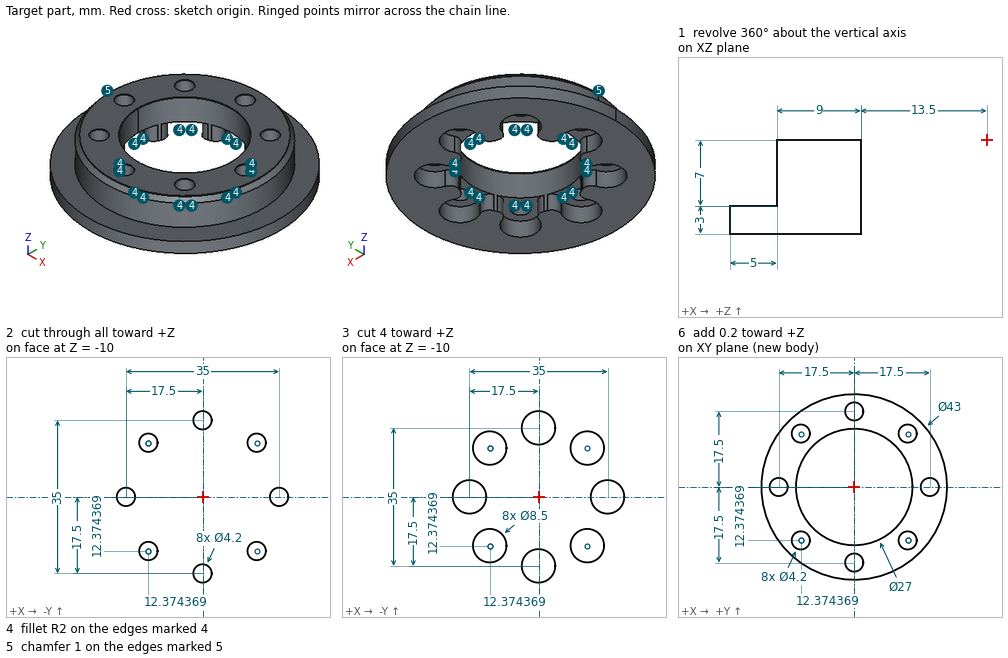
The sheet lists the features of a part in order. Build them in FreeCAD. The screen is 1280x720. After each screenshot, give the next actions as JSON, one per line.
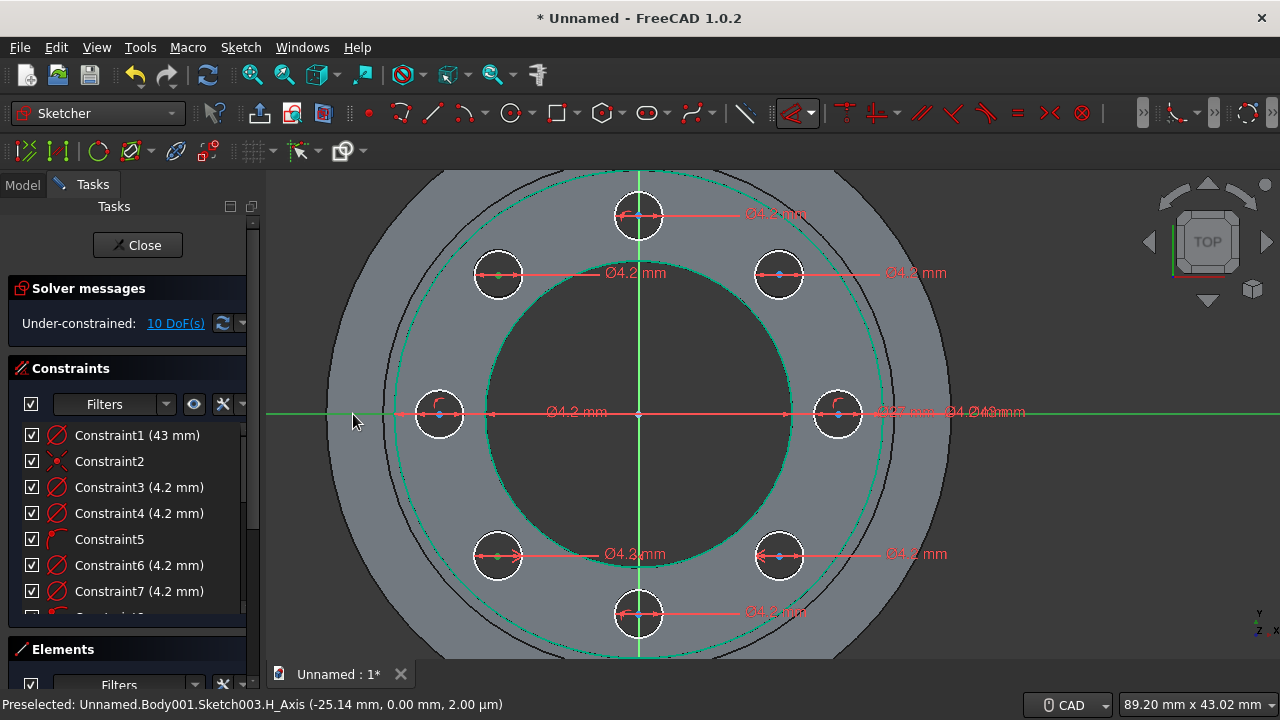
{"action": "key", "text": "s"}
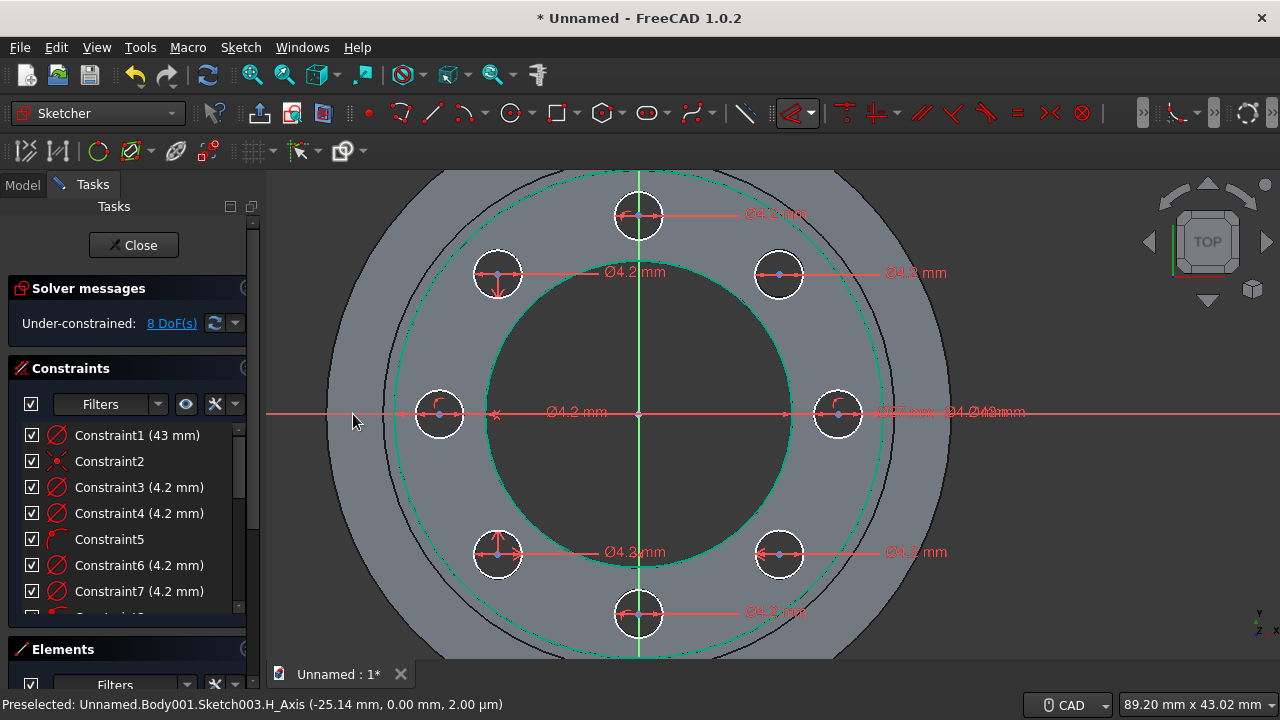
{"action": "left_click", "coordinate": [780, 554]}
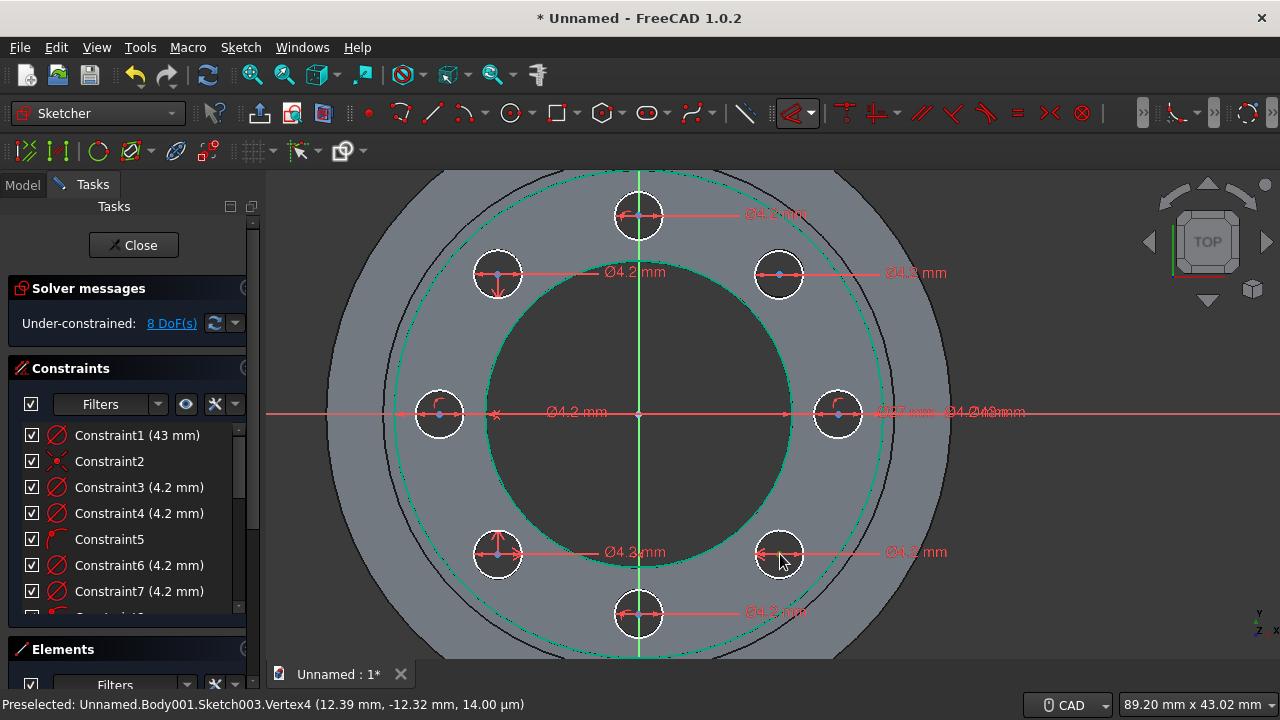
{"action": "left_click", "coordinate": [779, 275]}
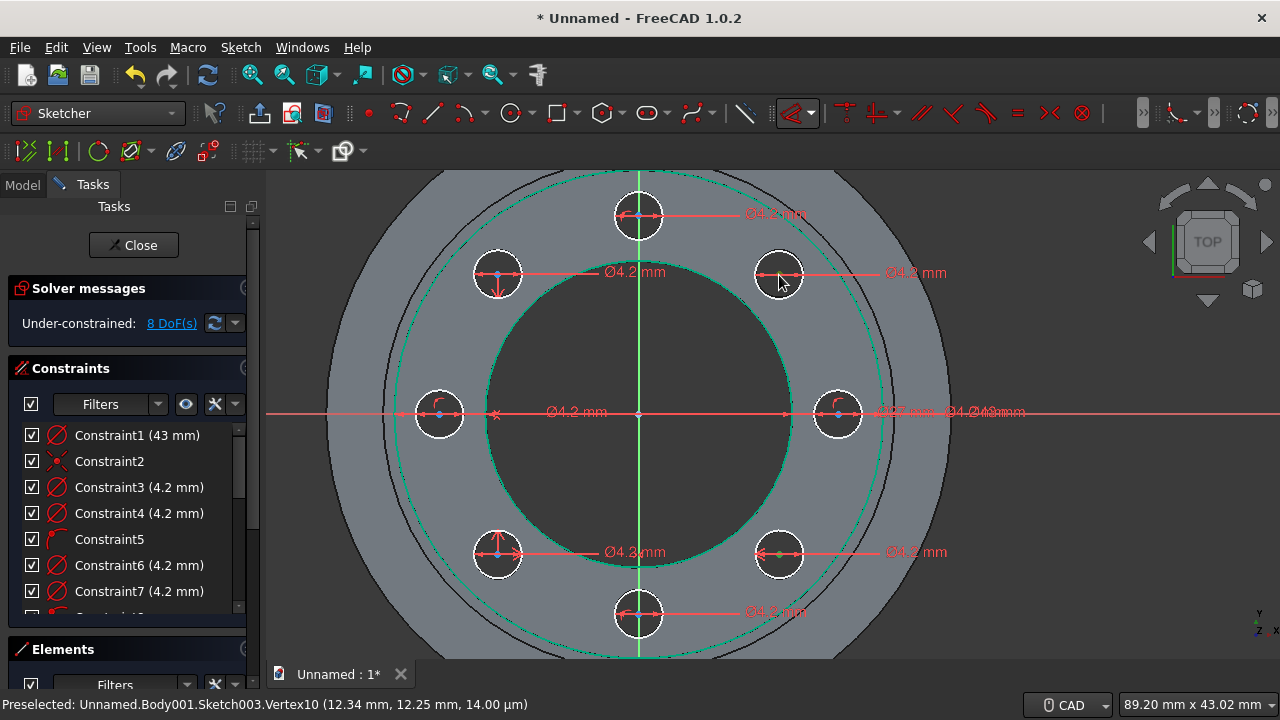
{"action": "left_click", "coordinate": [353, 414]}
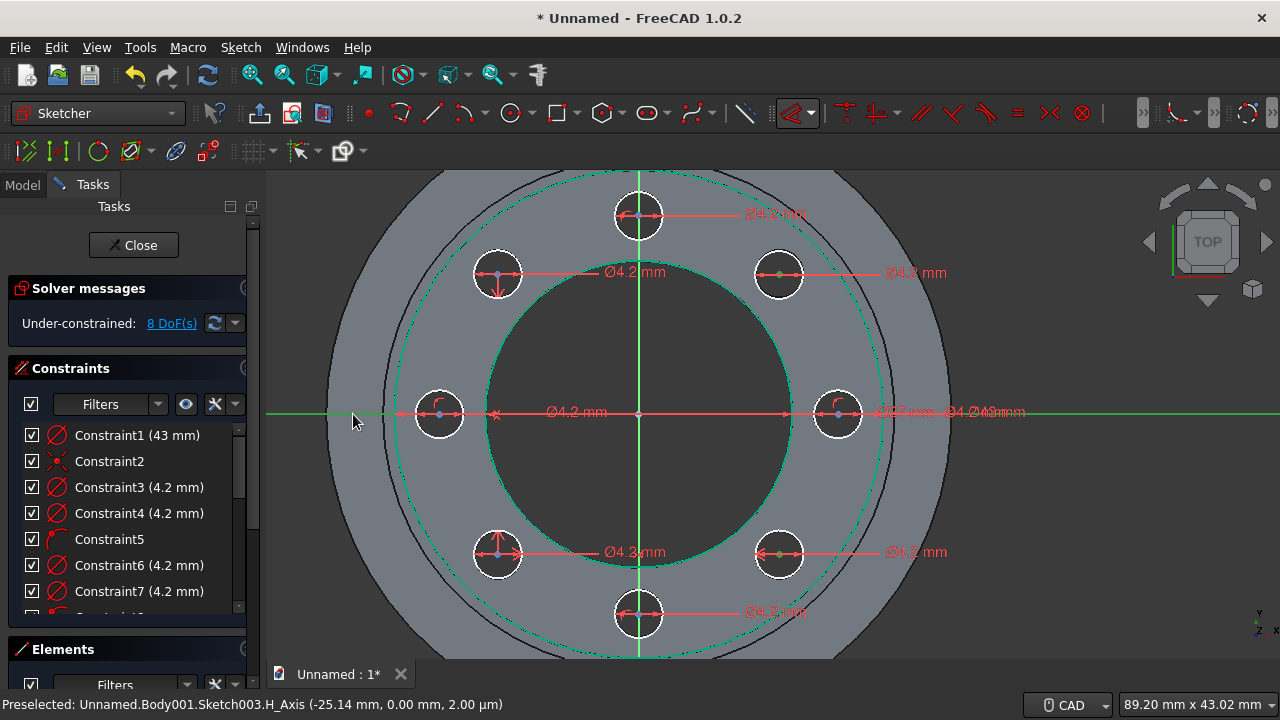
{"action": "left_click", "coordinate": [1050, 114]}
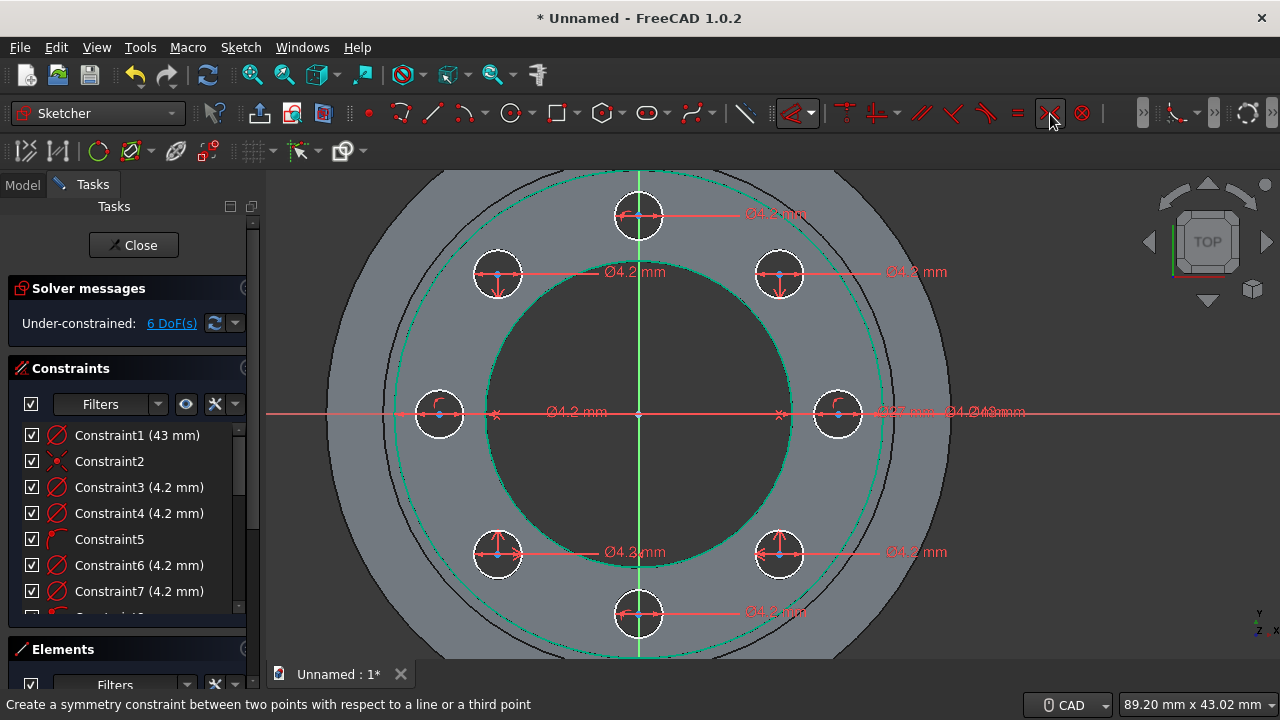
{"action": "left_click", "coordinate": [639, 614]}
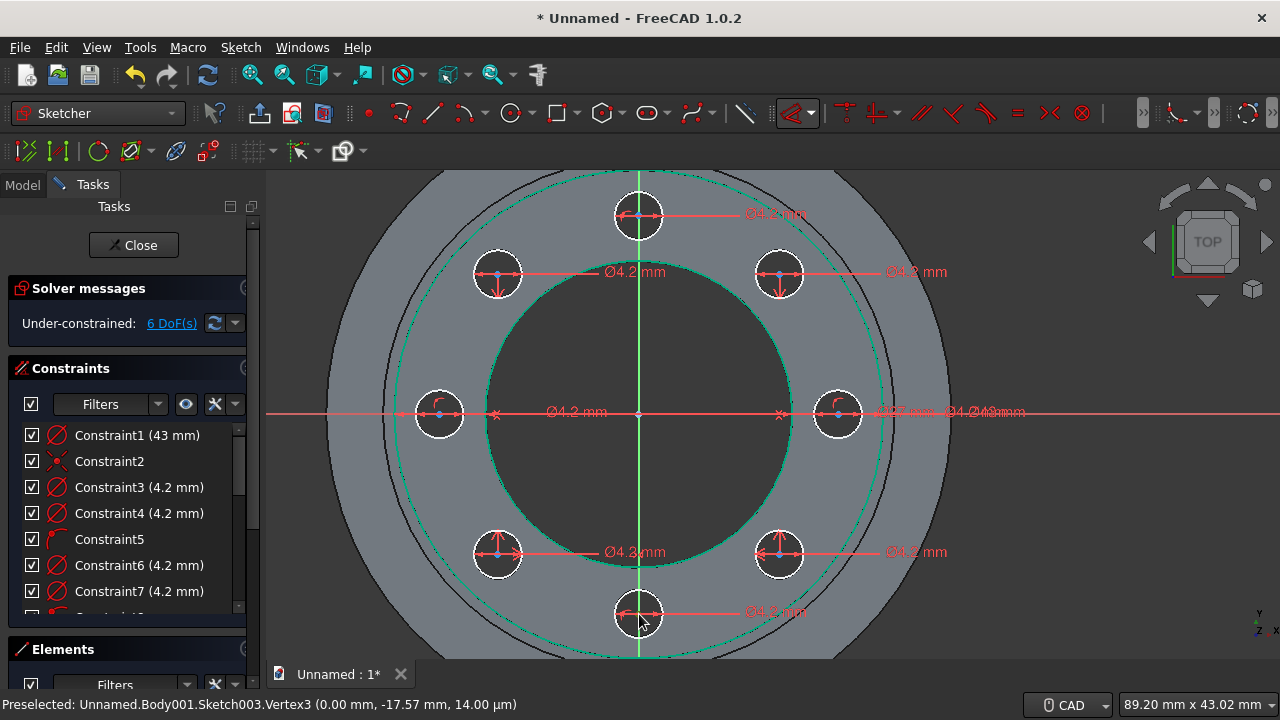
{"action": "key", "text": "i"}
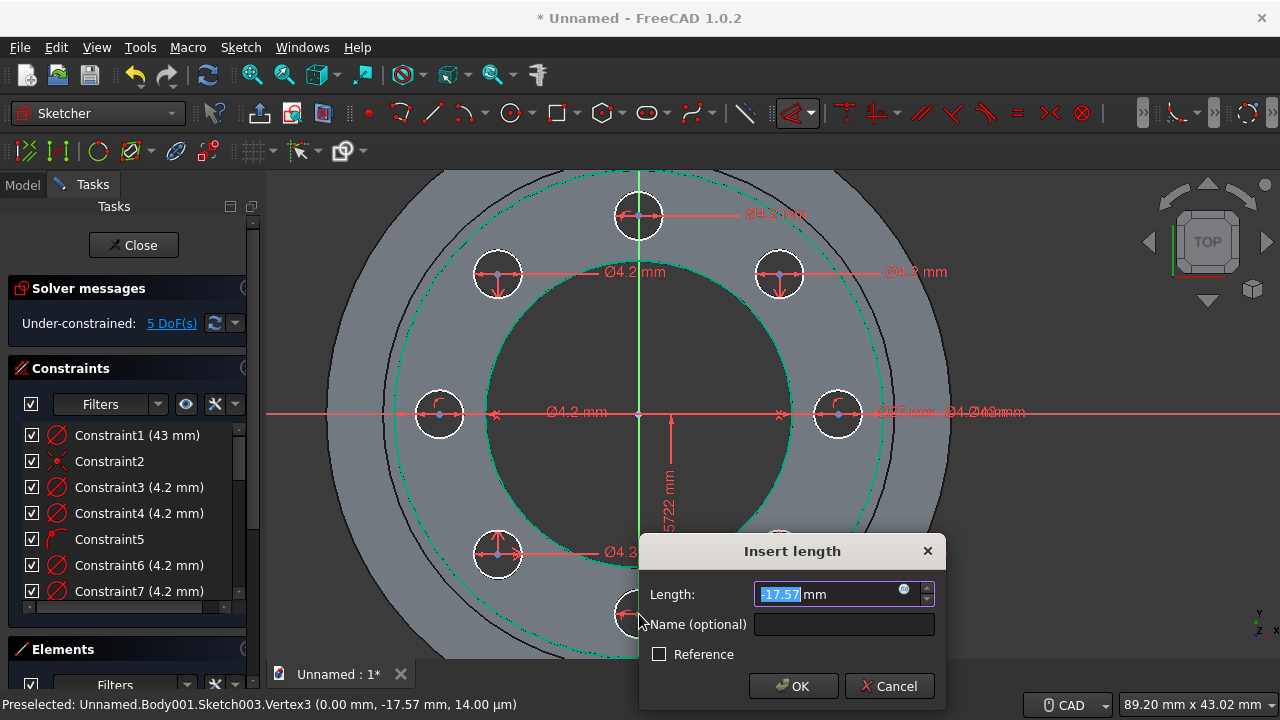
{"action": "type", "text": "-17.5"}
{"action": "key", "text": "Return"}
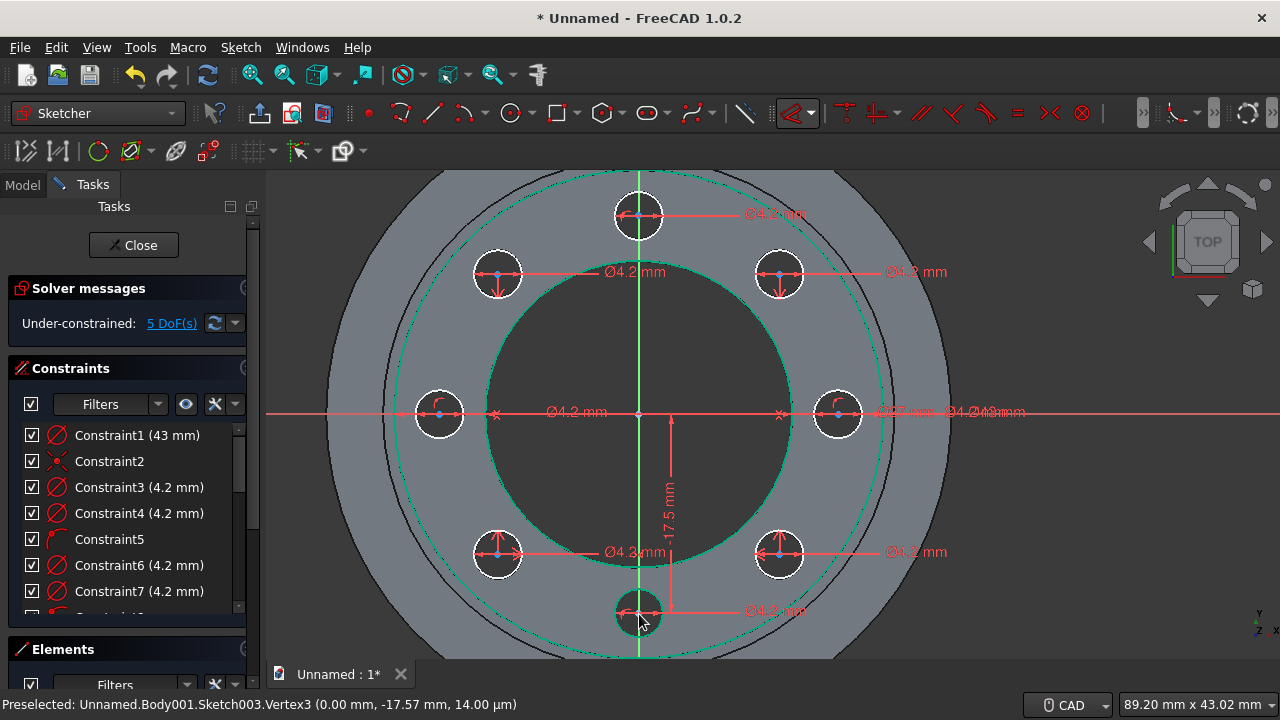
{"action": "left_click", "coordinate": [440, 414]}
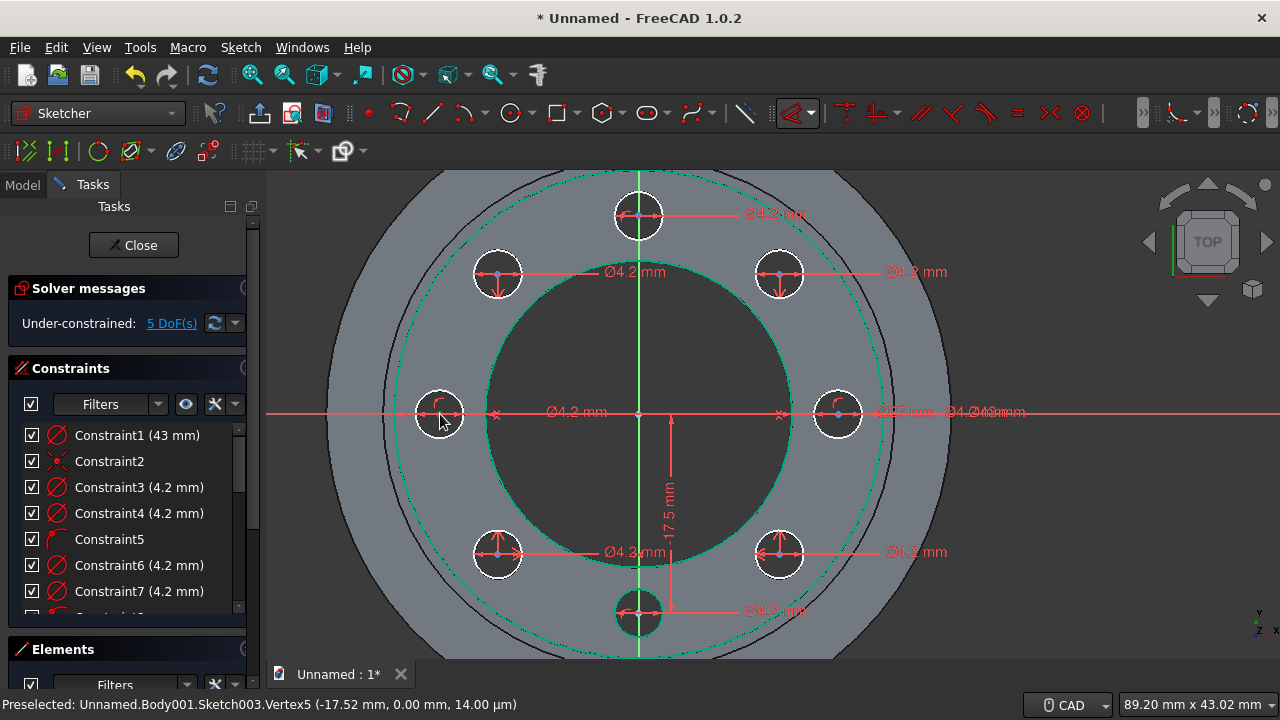
{"action": "left_click", "coordinate": [814, 114]}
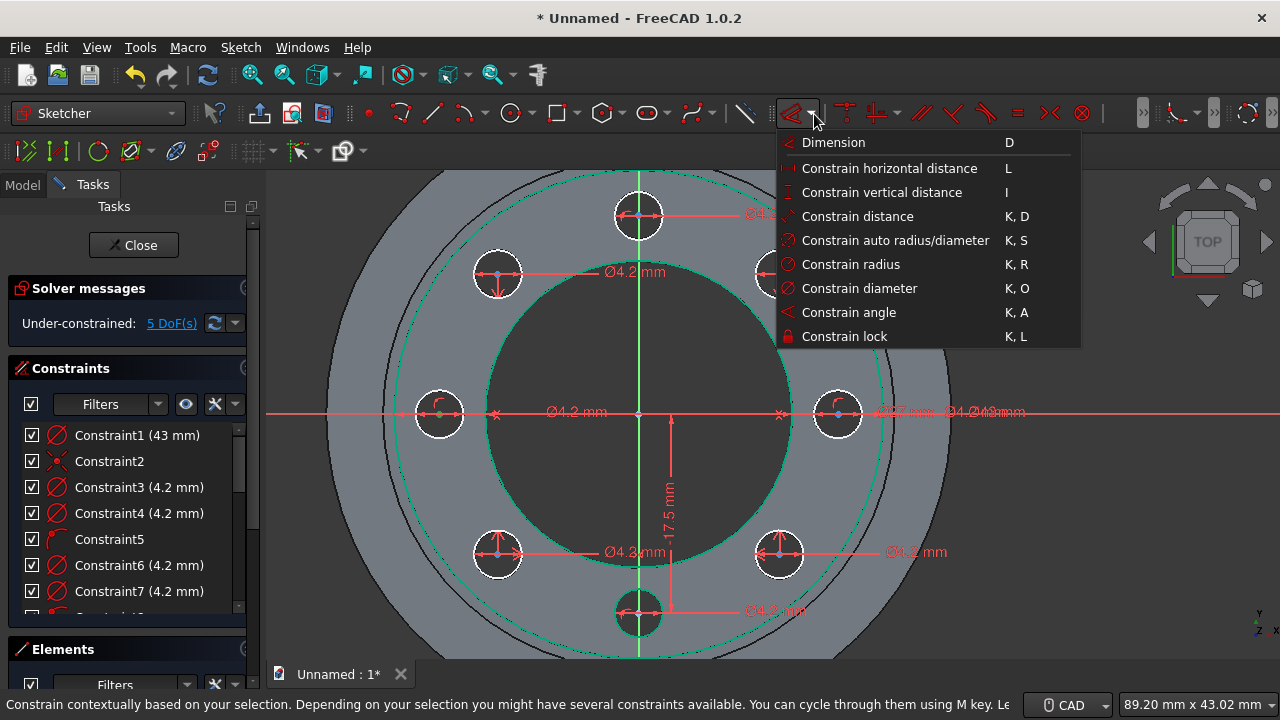
{"action": "left_click", "coordinate": [929, 168]}